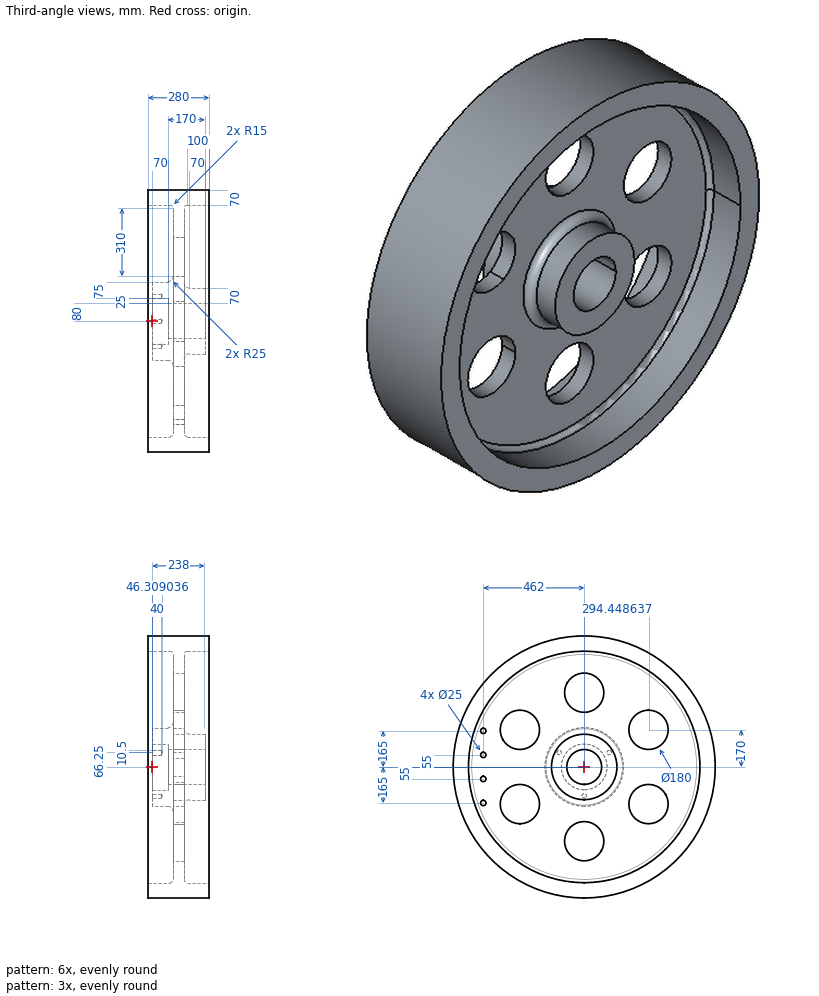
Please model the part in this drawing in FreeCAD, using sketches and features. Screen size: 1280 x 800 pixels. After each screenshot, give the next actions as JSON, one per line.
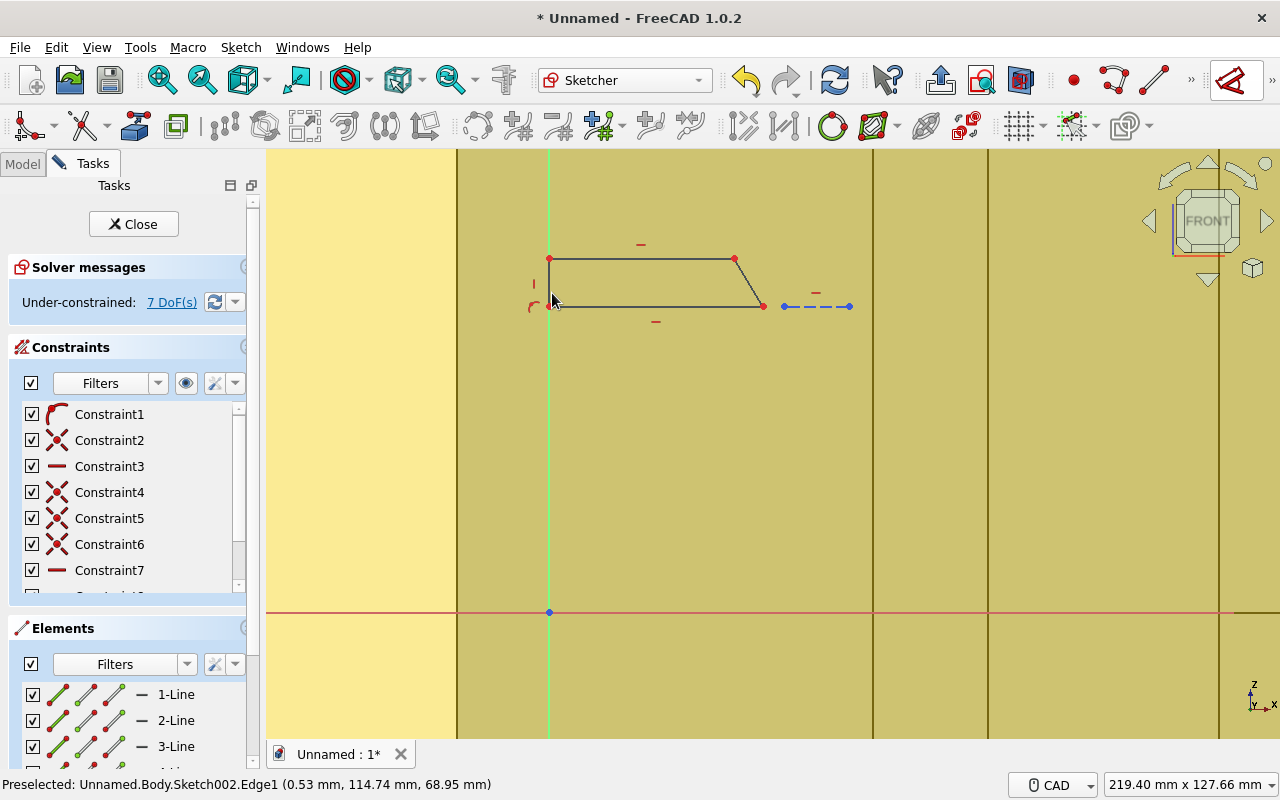
{"action": "left_click", "coordinate": [605, 259]}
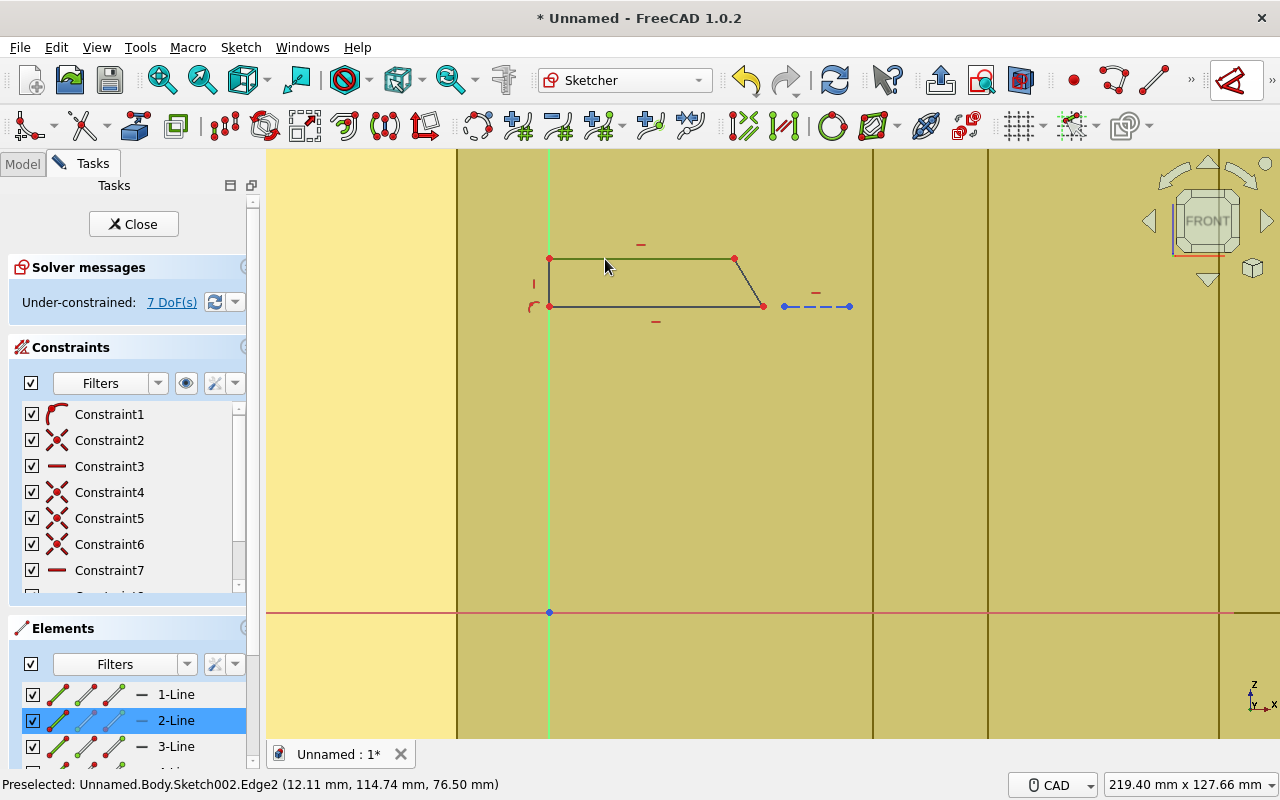
{"action": "key", "text": "l"}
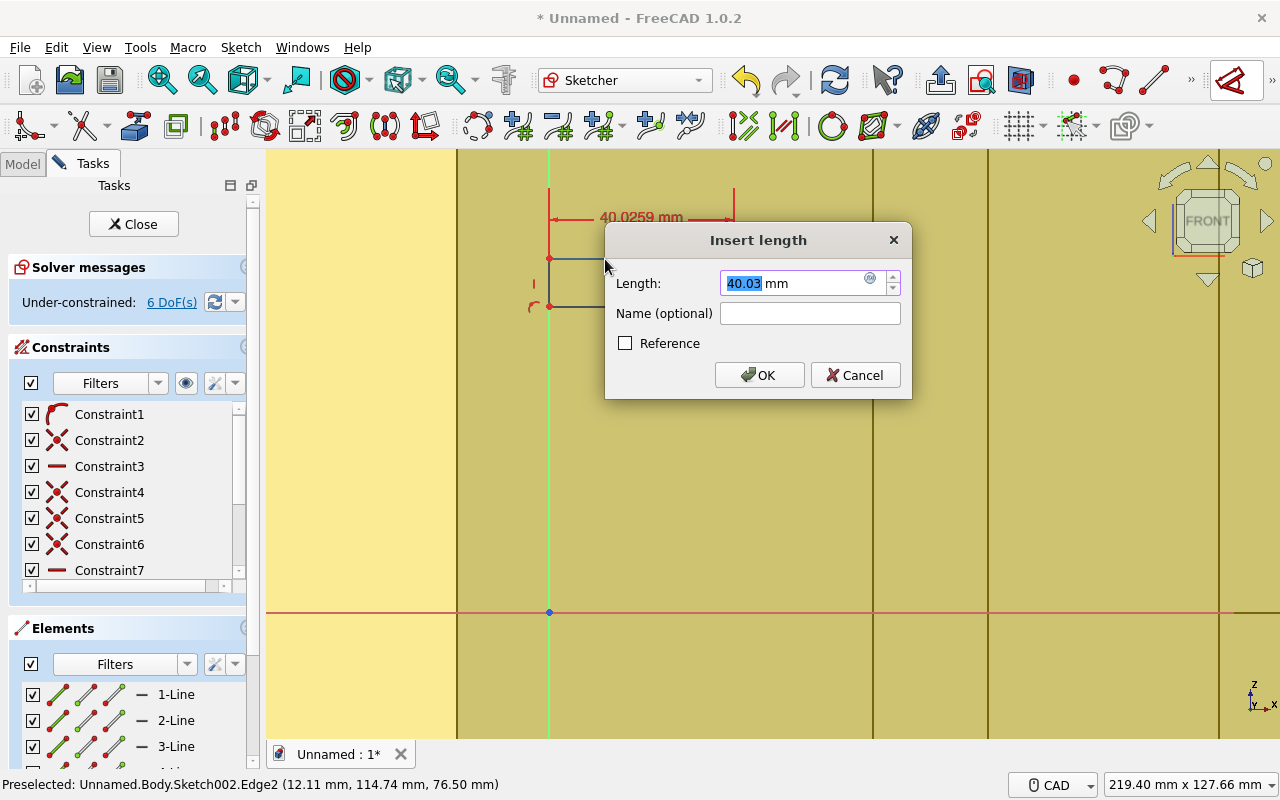
{"action": "type", "text": "40"}
{"action": "key", "text": "Return"}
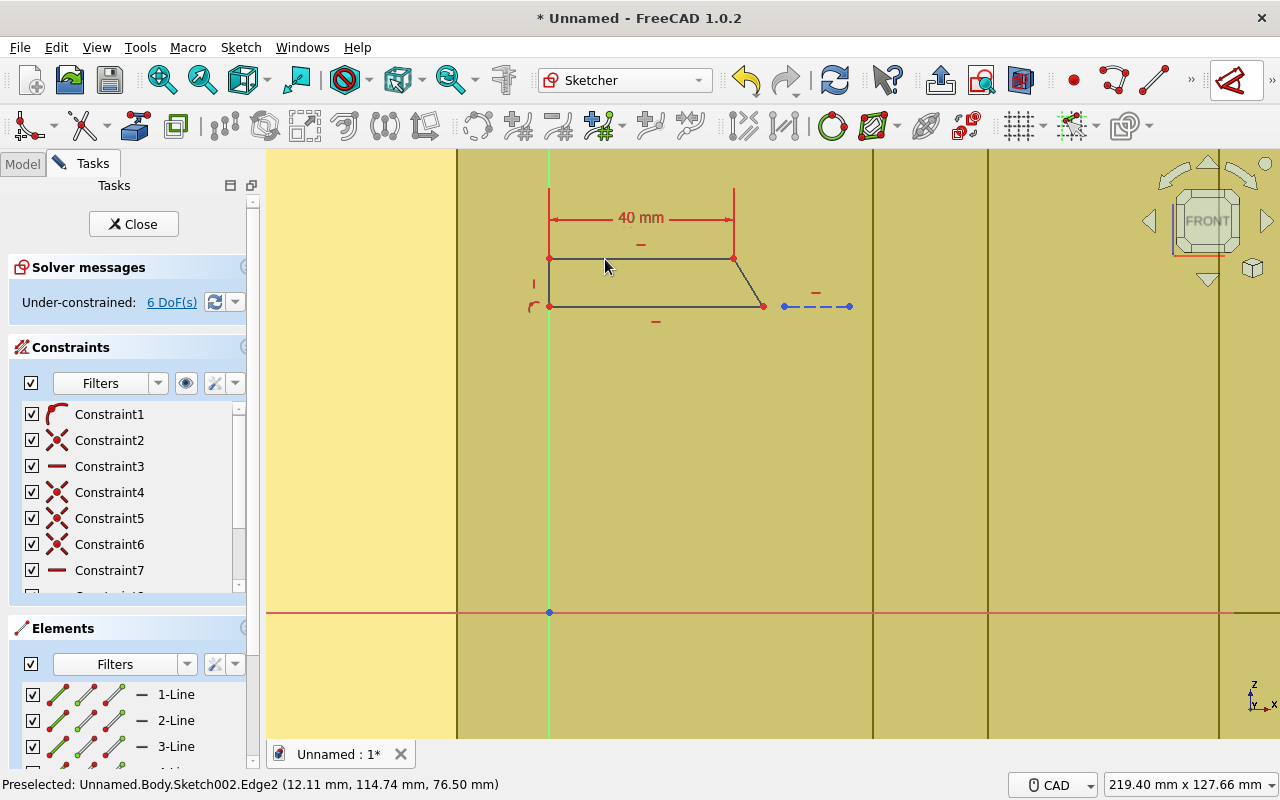
{"action": "left_click", "coordinate": [549, 293]}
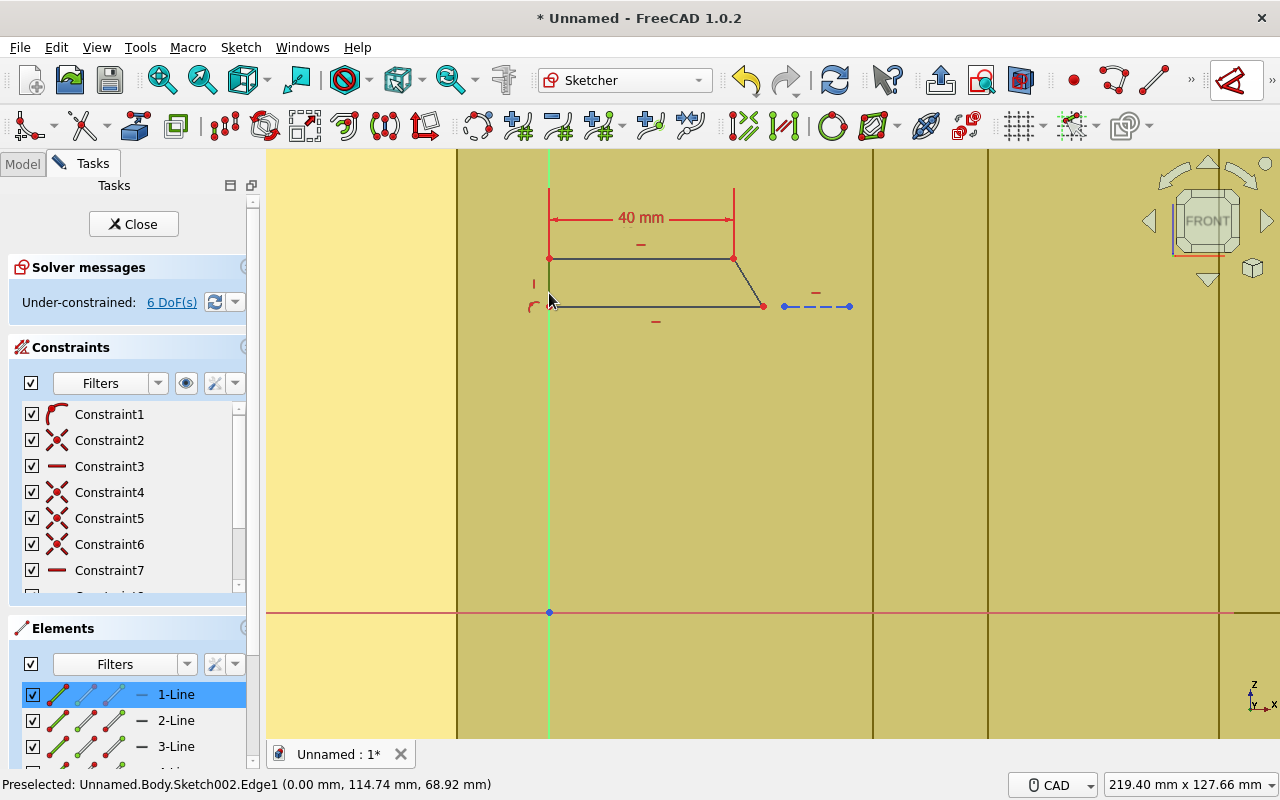
{"action": "key", "text": "i"}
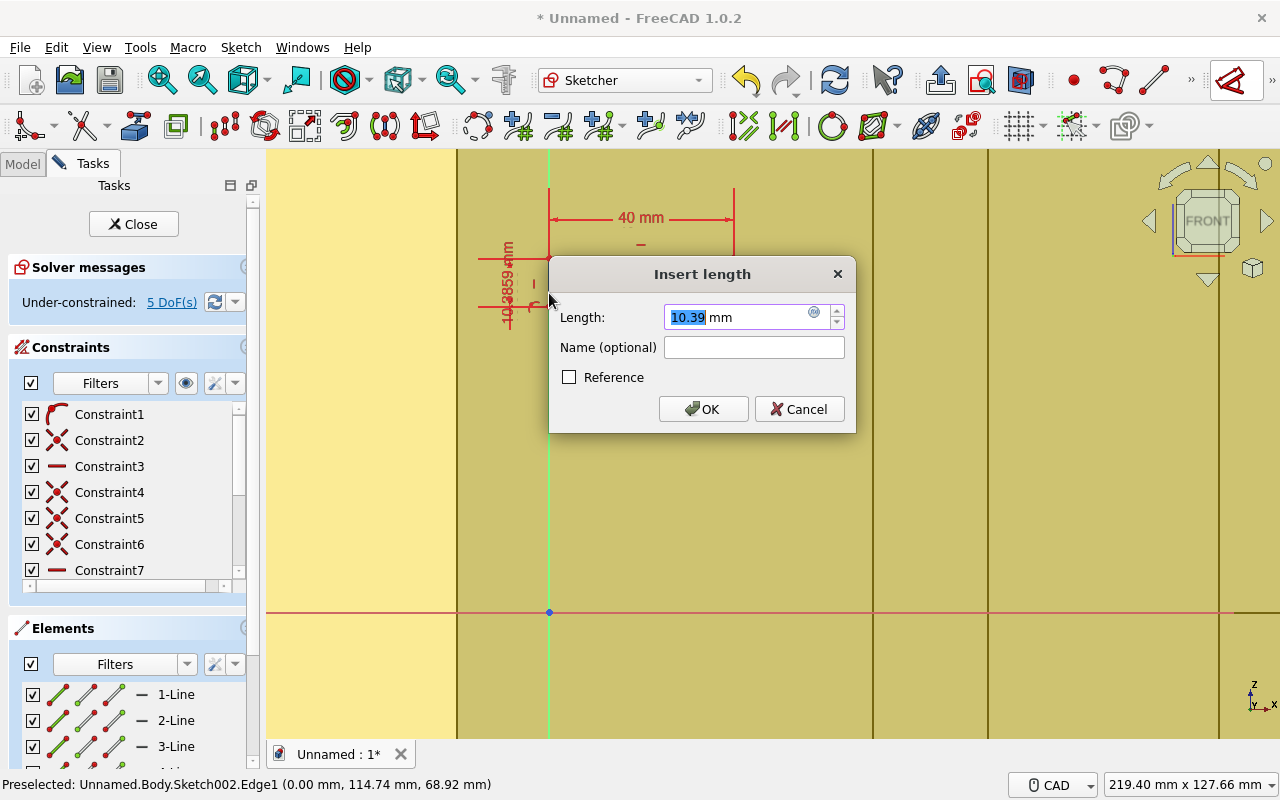
{"action": "type", "text": "10.5"}
{"action": "key", "text": "Return"}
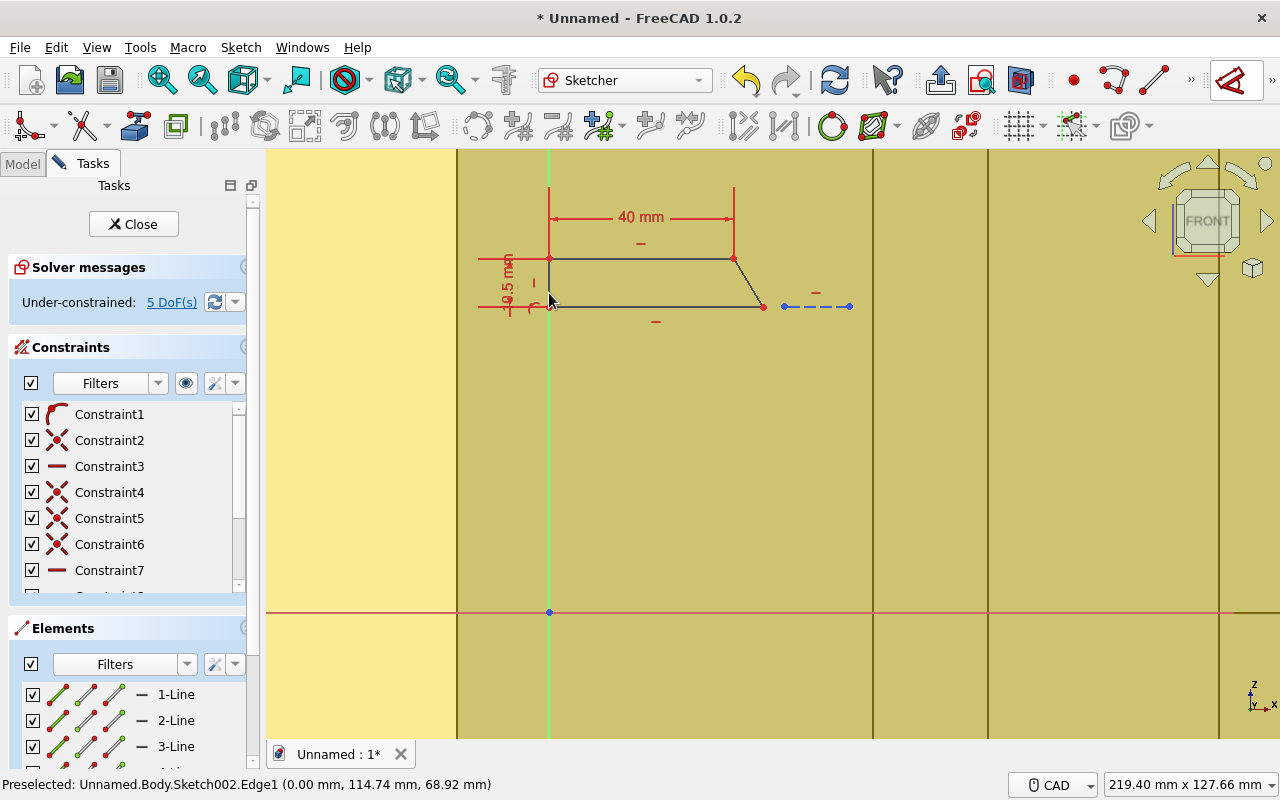
{"action": "left_click", "coordinate": [549, 307]}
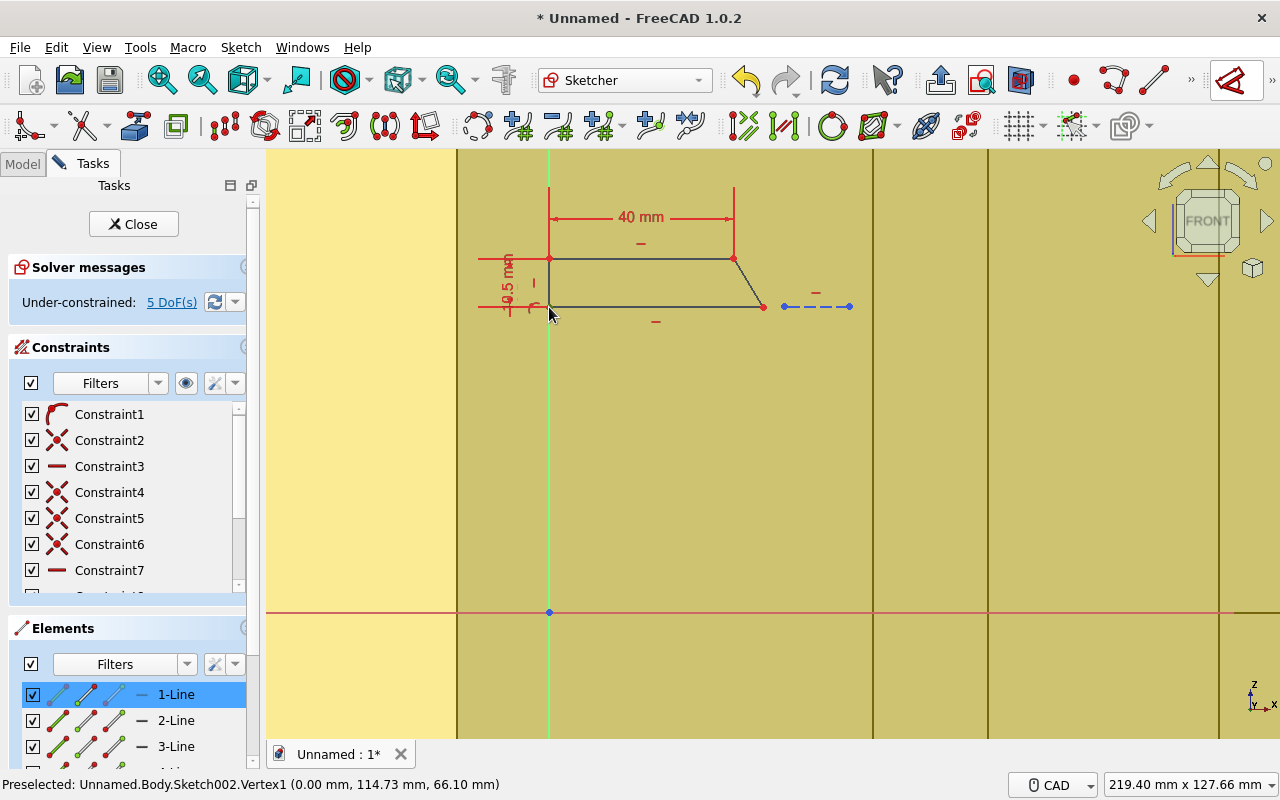
{"action": "left_click", "coordinate": [1258, 80]}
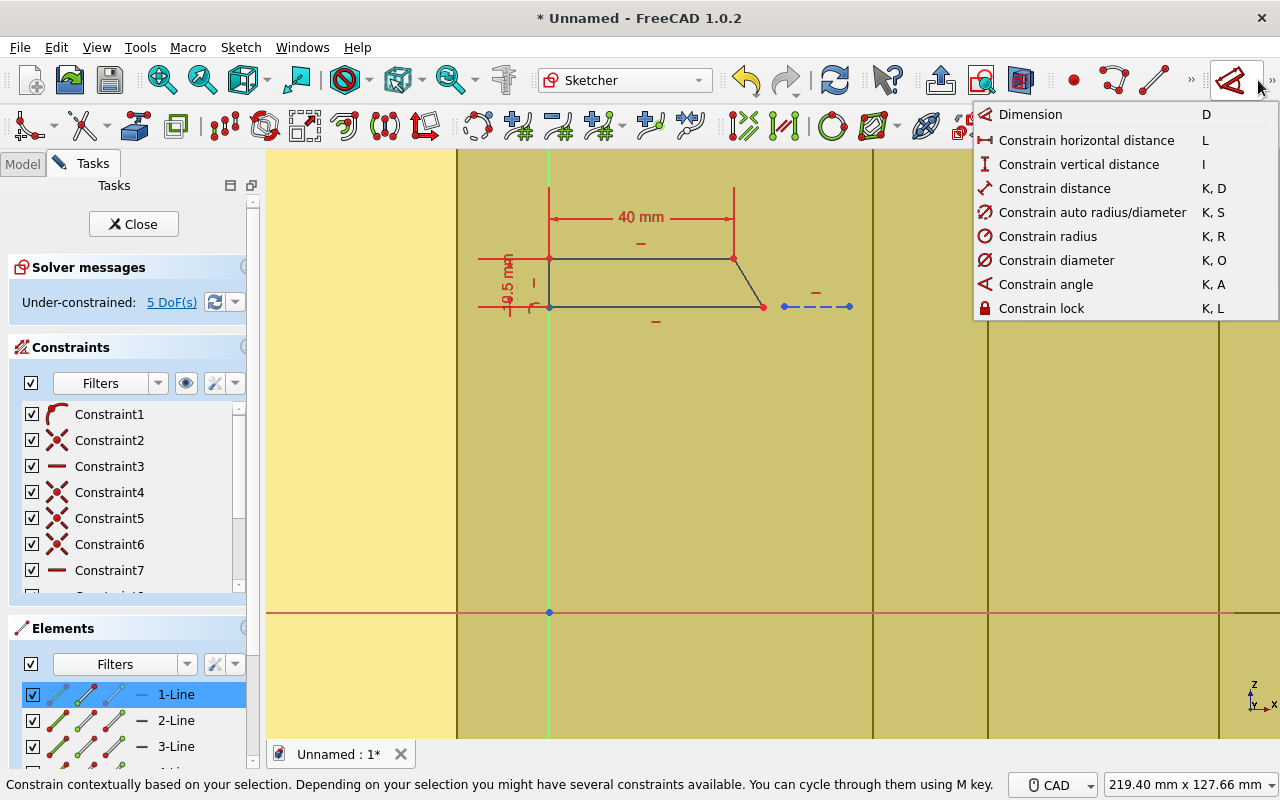
{"action": "left_click", "coordinate": [1126, 164]}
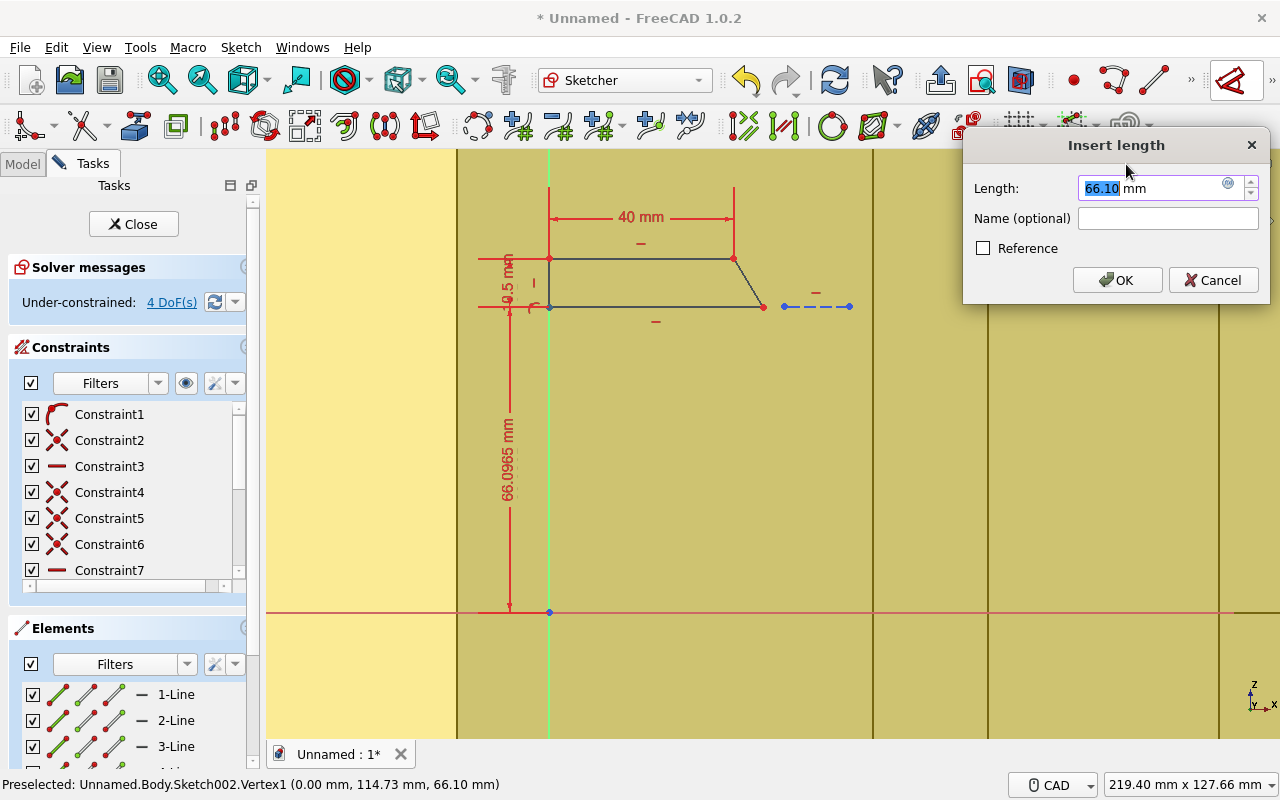
{"action": "type", "text": "66.25"}
{"action": "key", "text": "Return"}